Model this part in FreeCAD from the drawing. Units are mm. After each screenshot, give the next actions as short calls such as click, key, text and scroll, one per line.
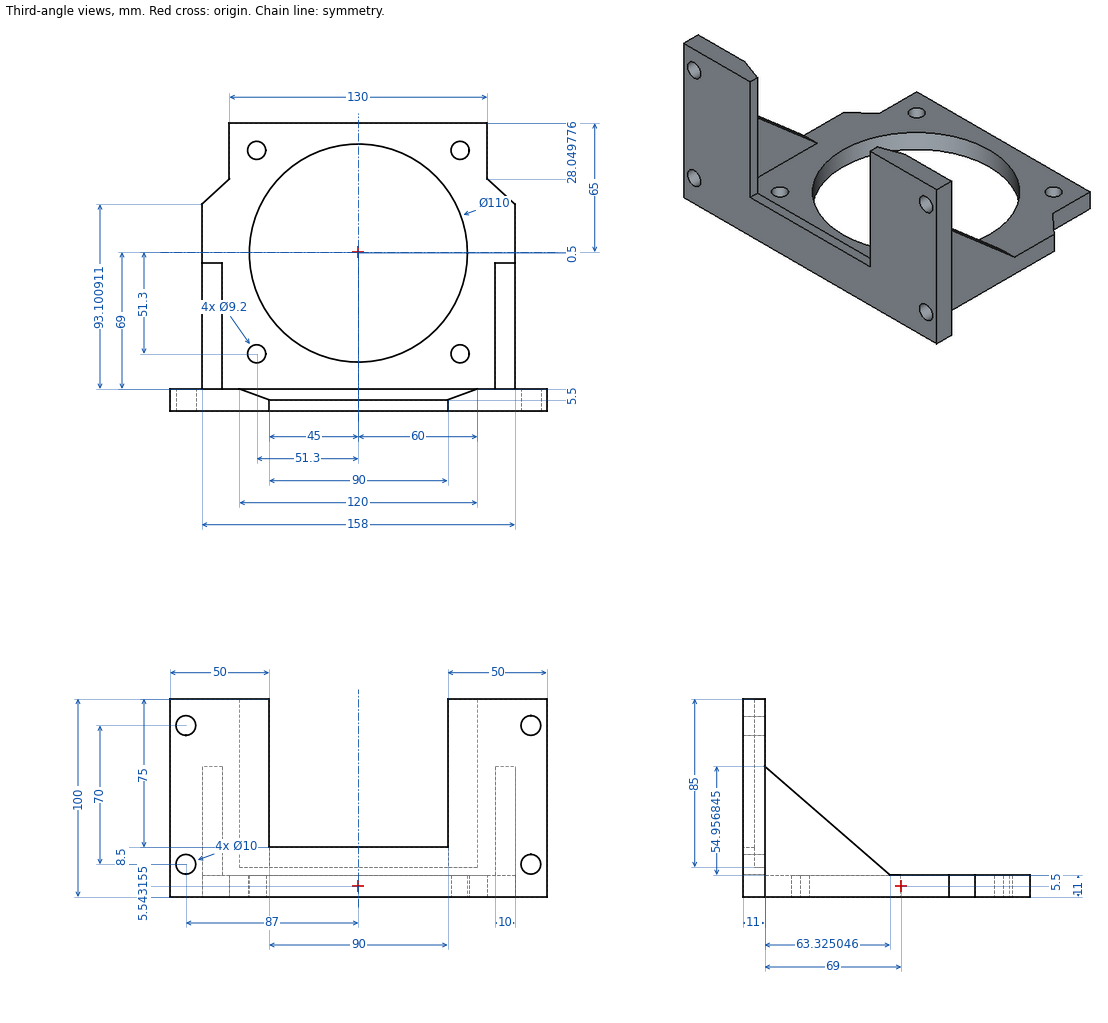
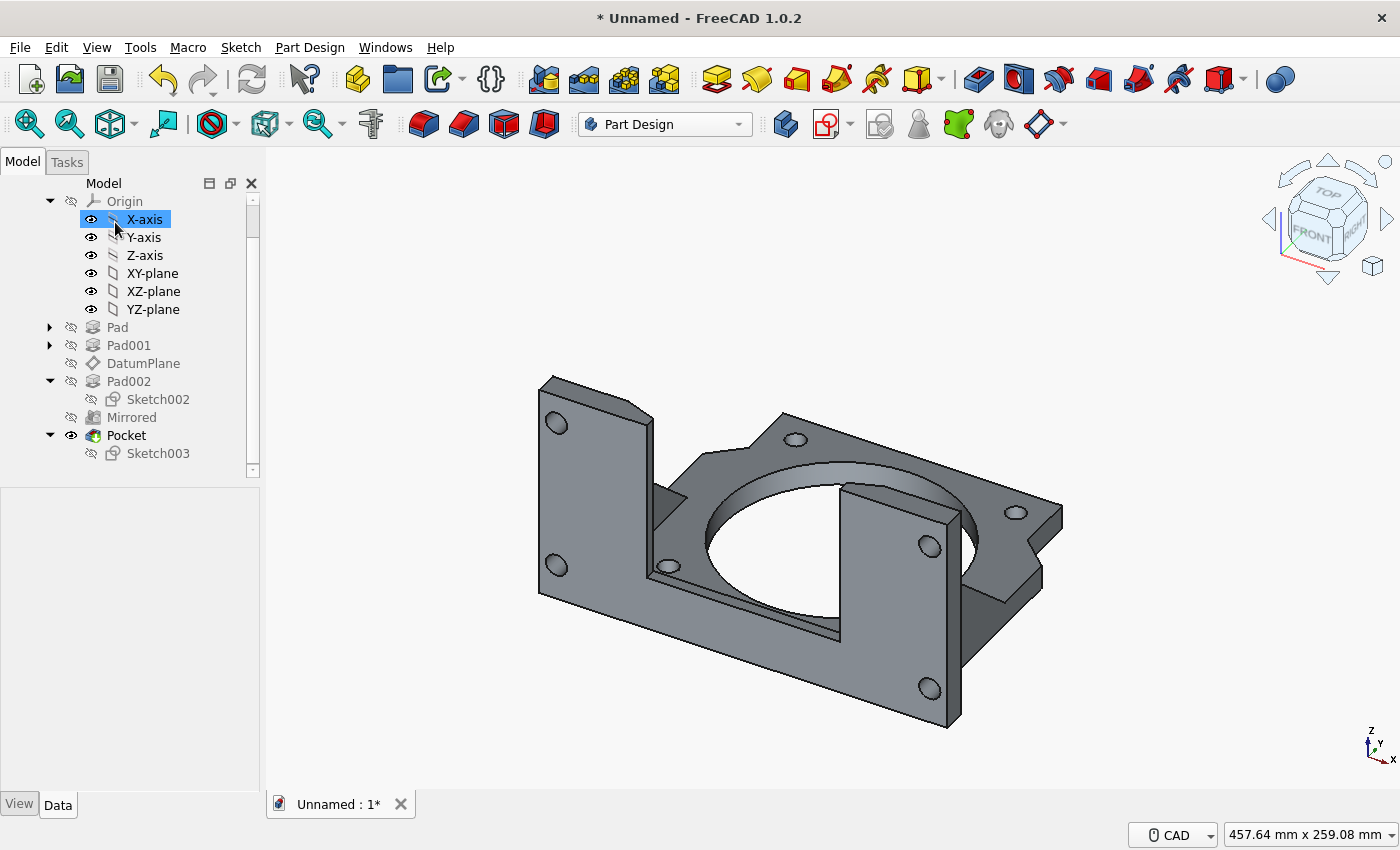
key(0)